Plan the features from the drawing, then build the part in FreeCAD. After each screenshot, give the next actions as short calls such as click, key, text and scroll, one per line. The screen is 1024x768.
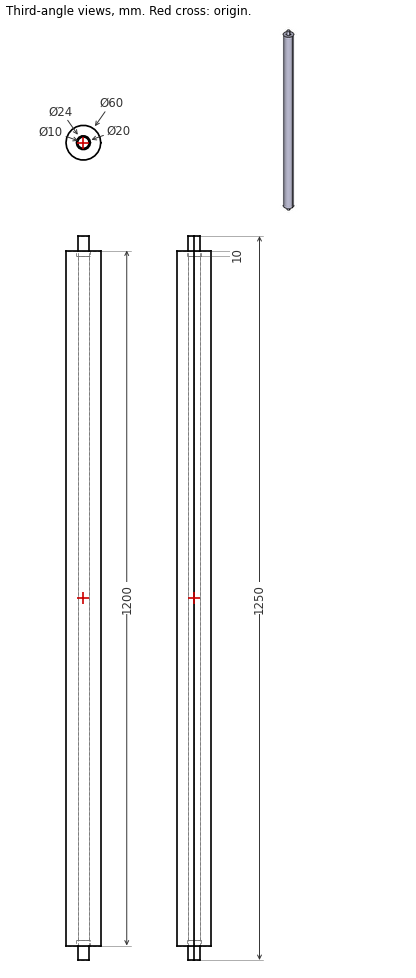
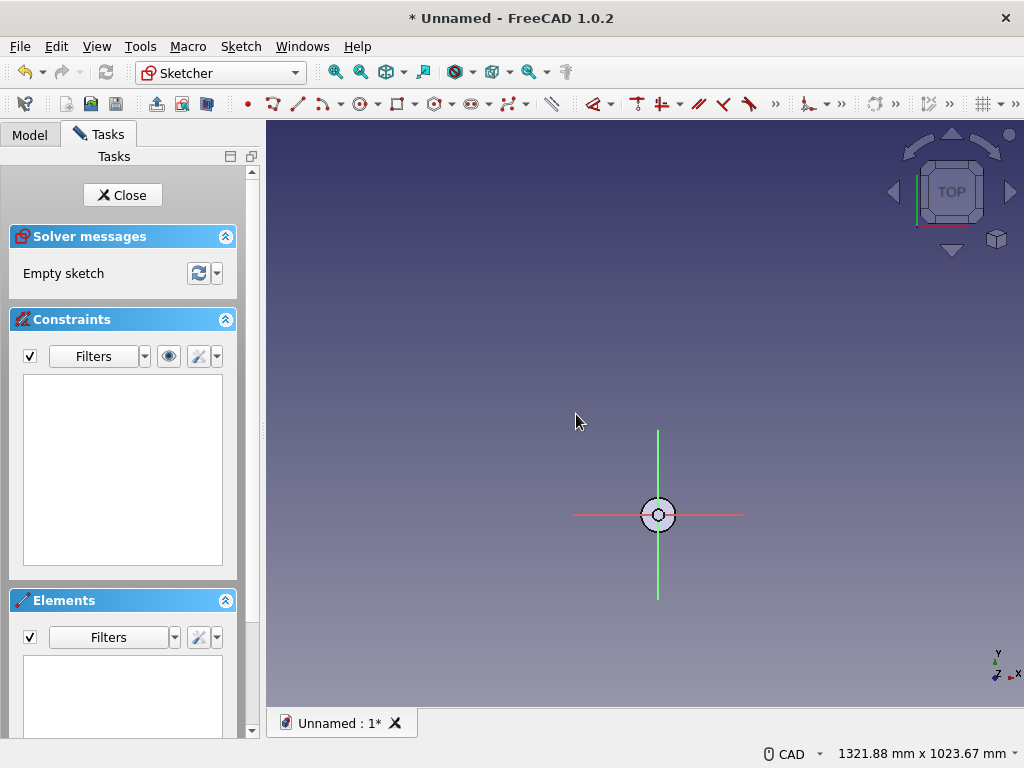
scroll(663, 520, up, 15)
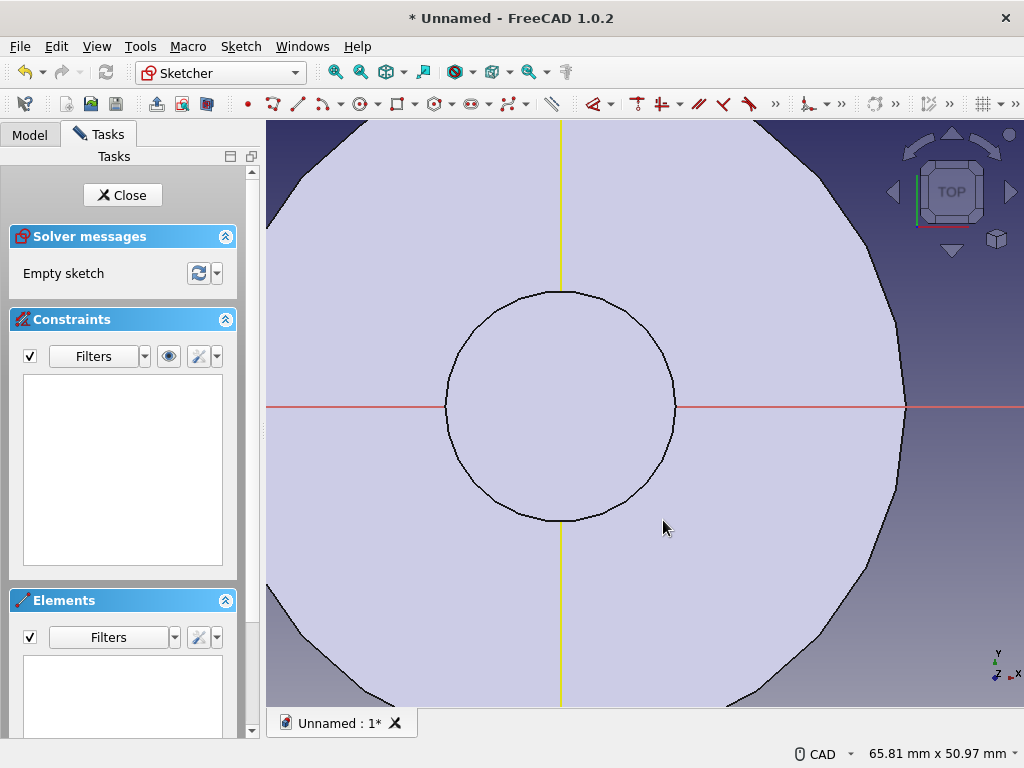
scroll(528, 392, up, 2)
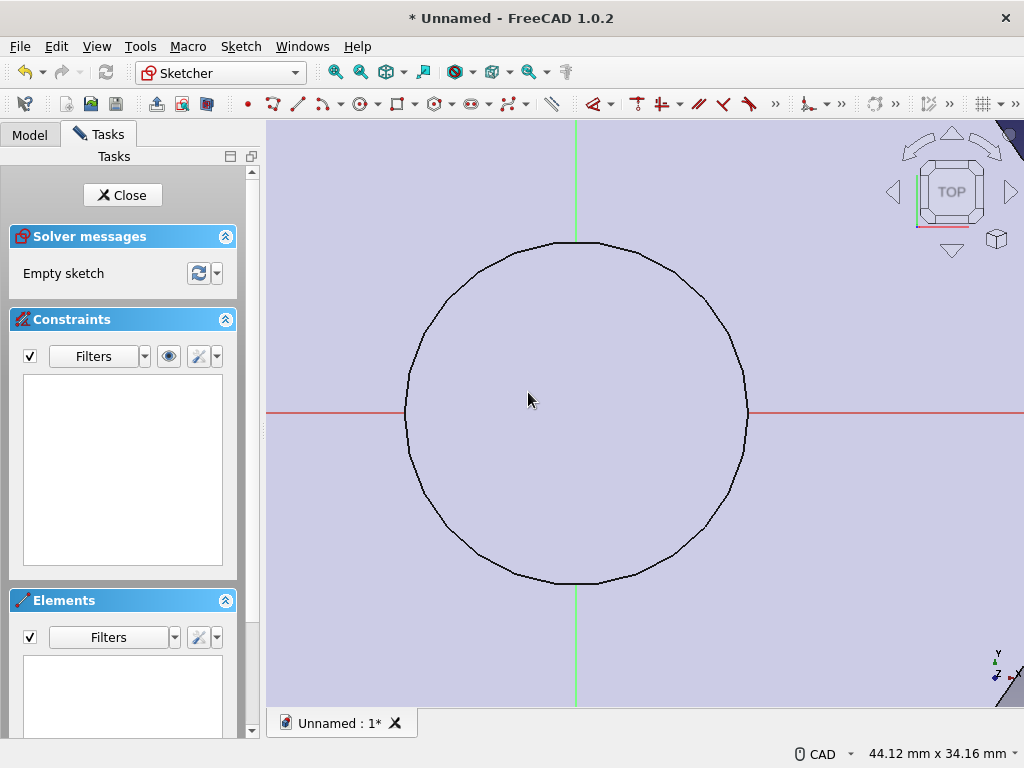
click(360, 104)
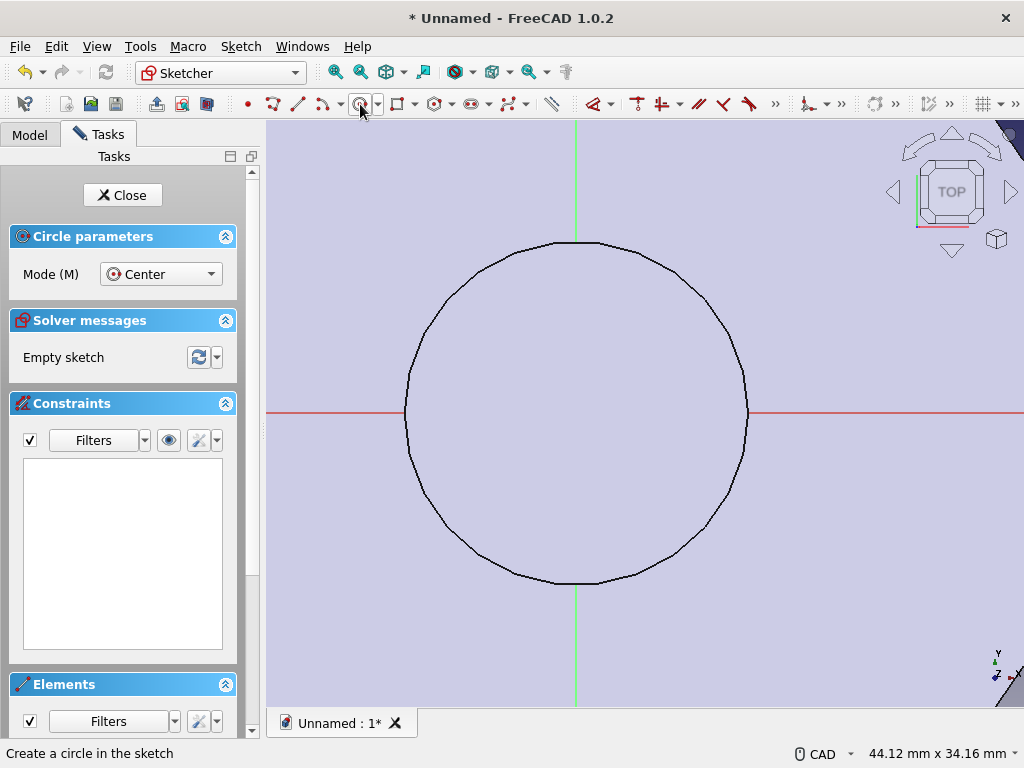
click(576, 413)
click(722, 268)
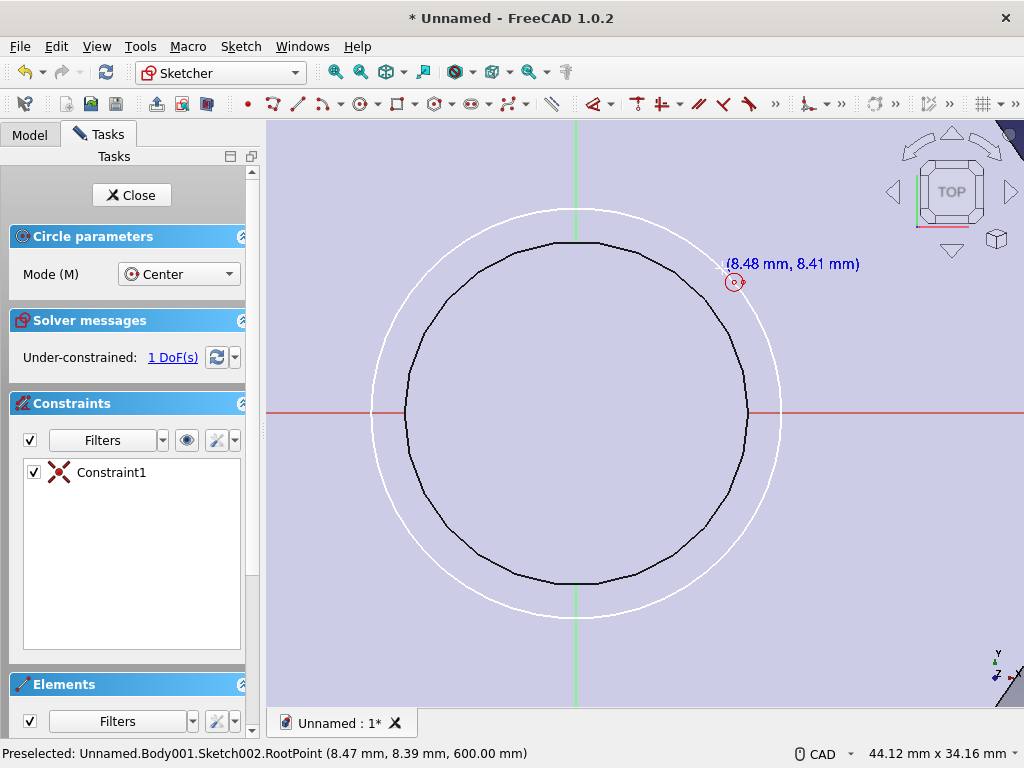
click(576, 413)
click(637, 353)
key(Escape)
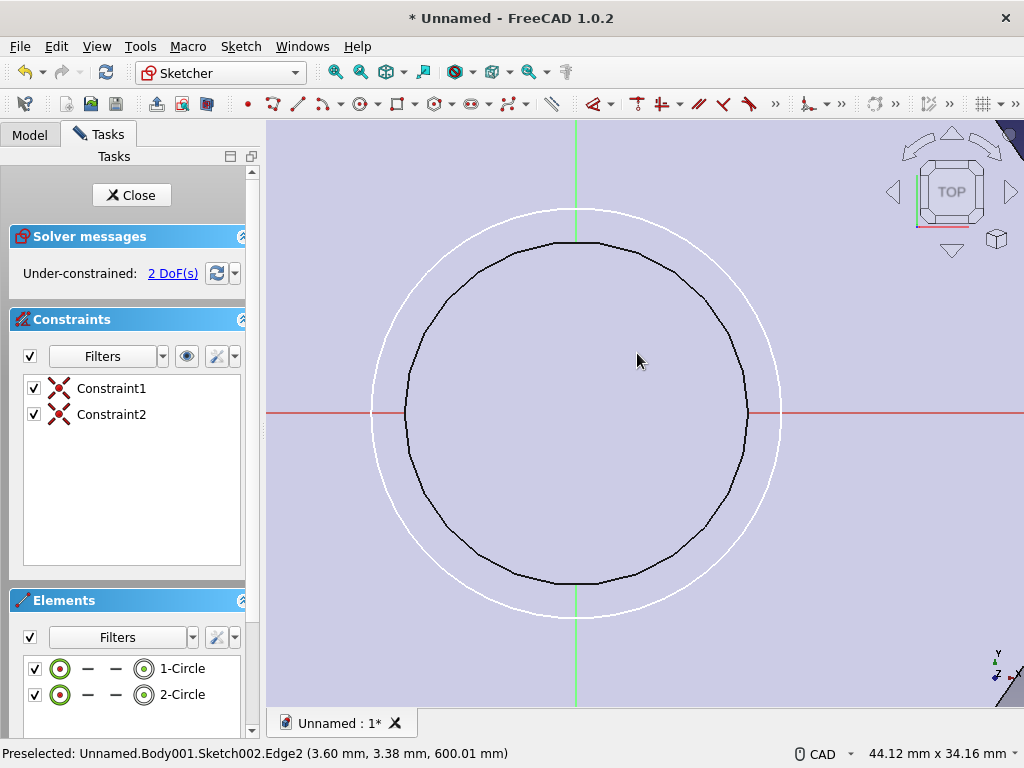
key(d)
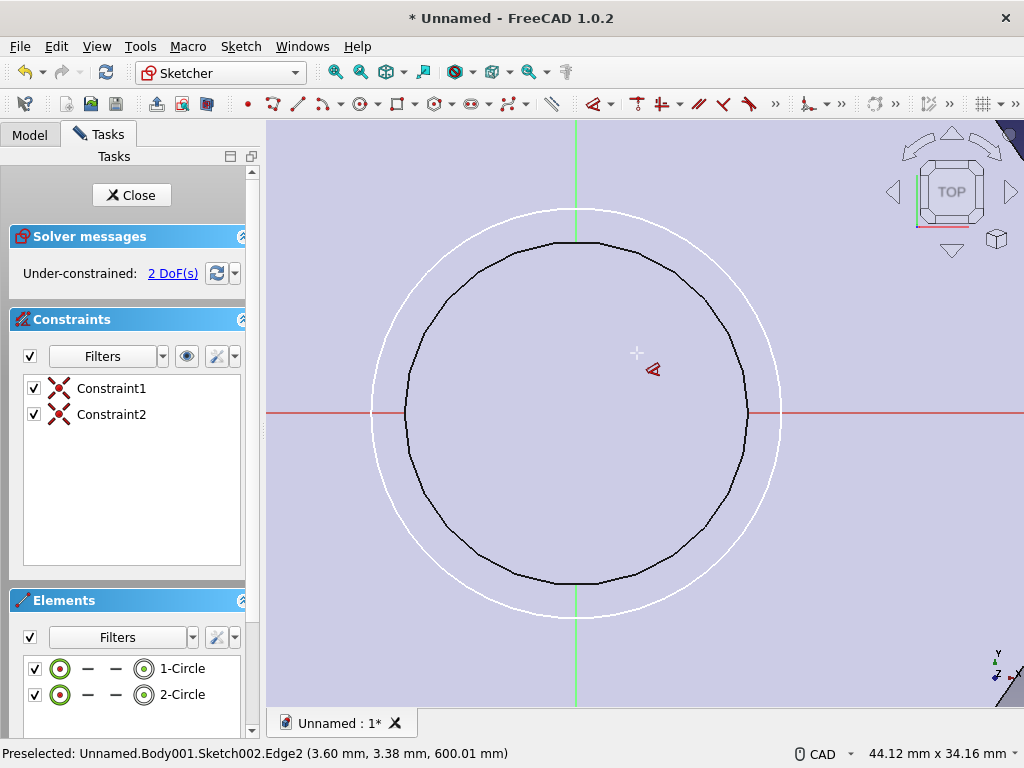
click(721, 268)
click(744, 245)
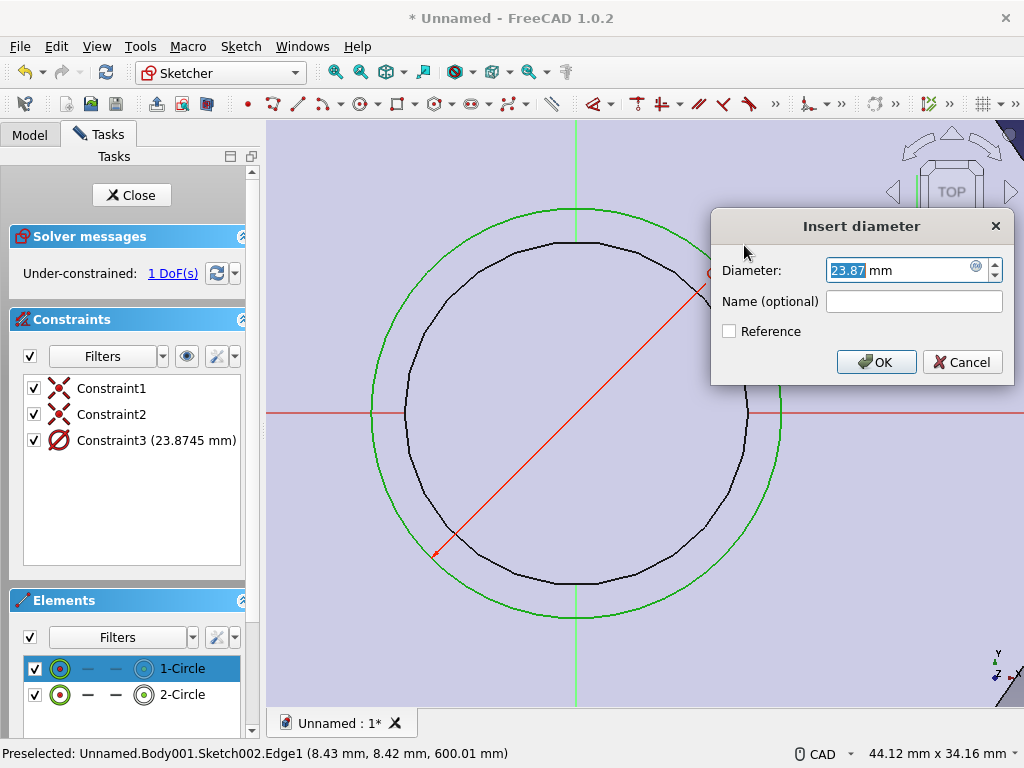
text(24)
key(Return)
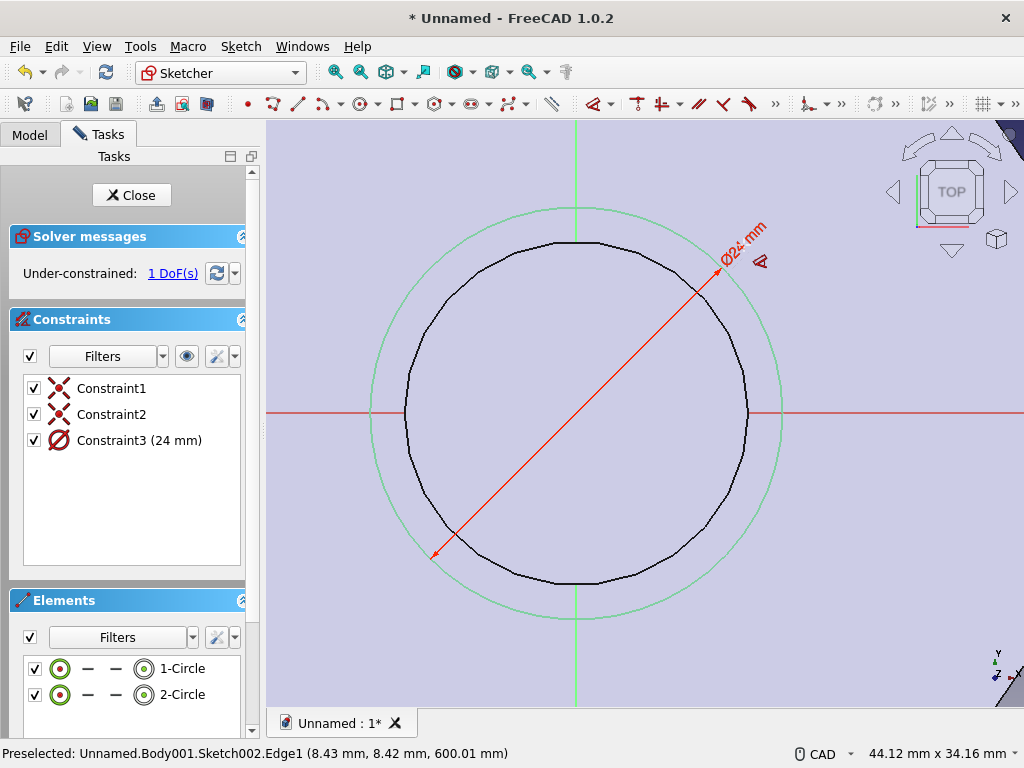
click(636, 353)
click(658, 330)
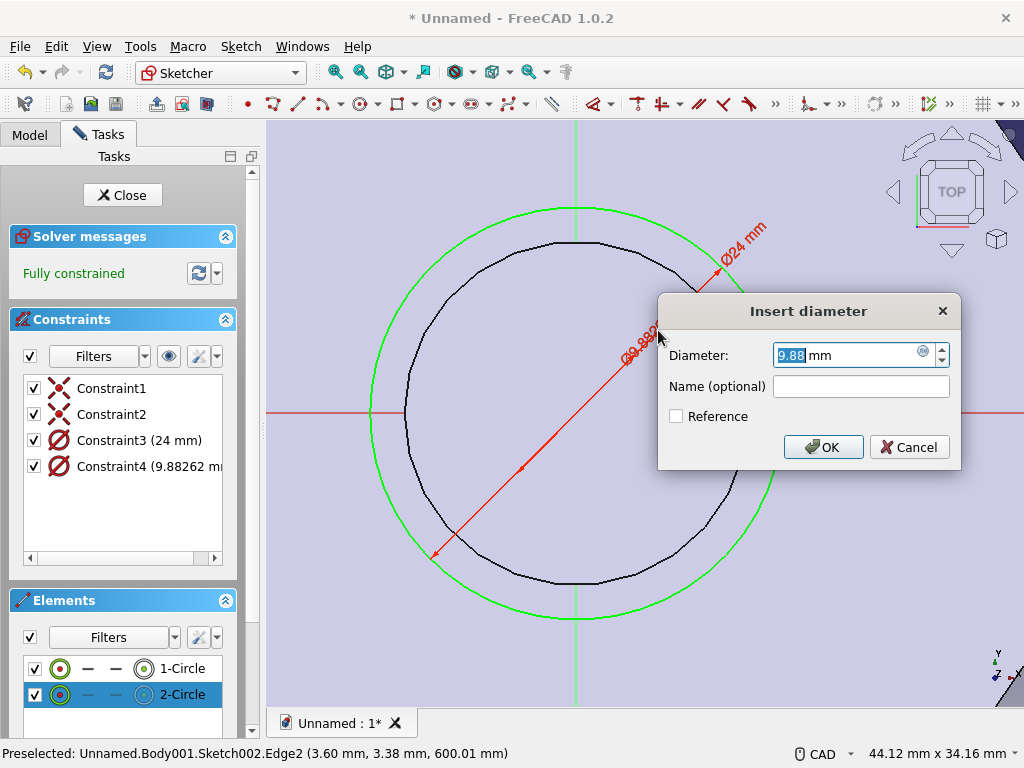
text(10)
key(Return)
key(Escape)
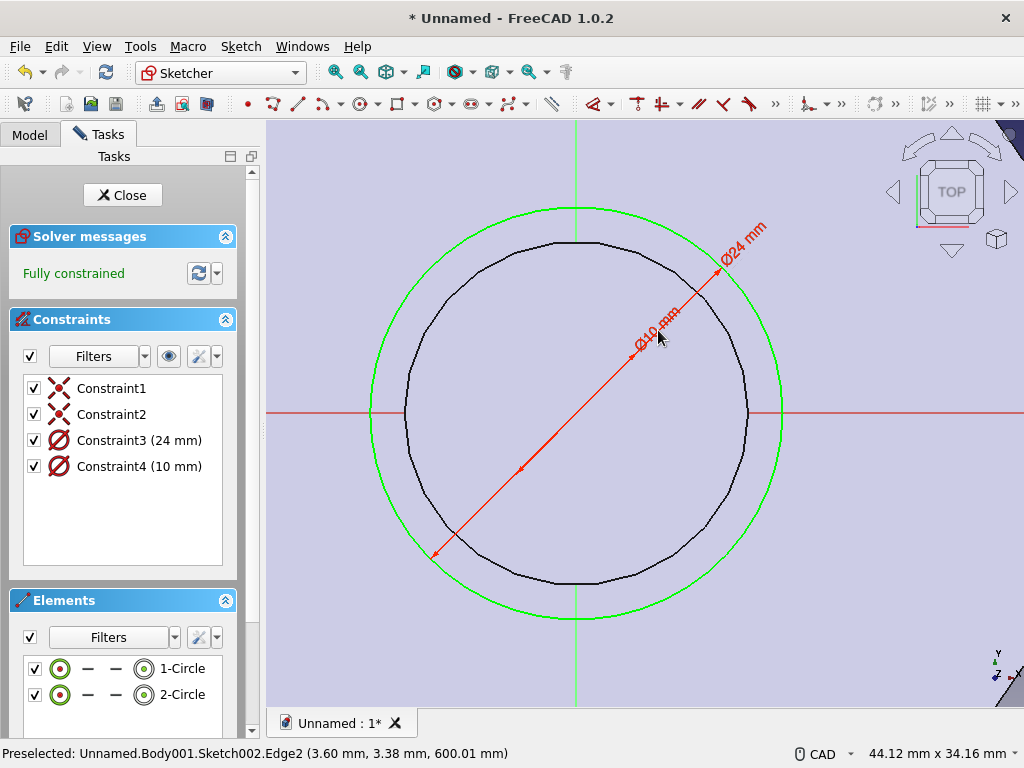
click(123, 195)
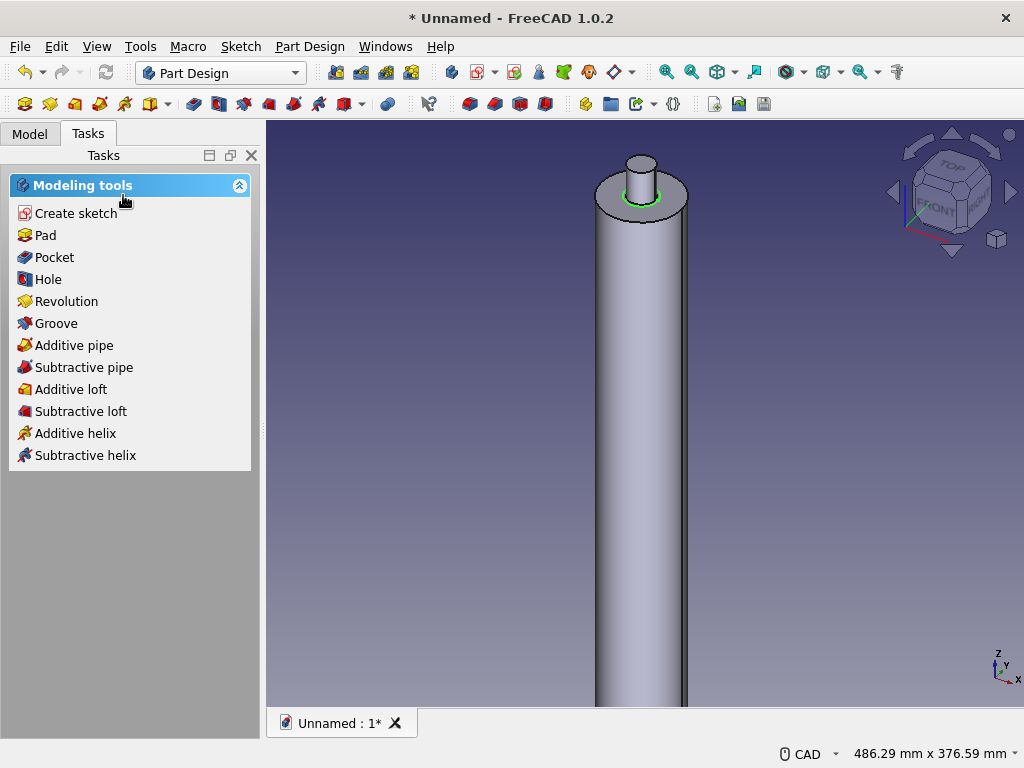
click(194, 104)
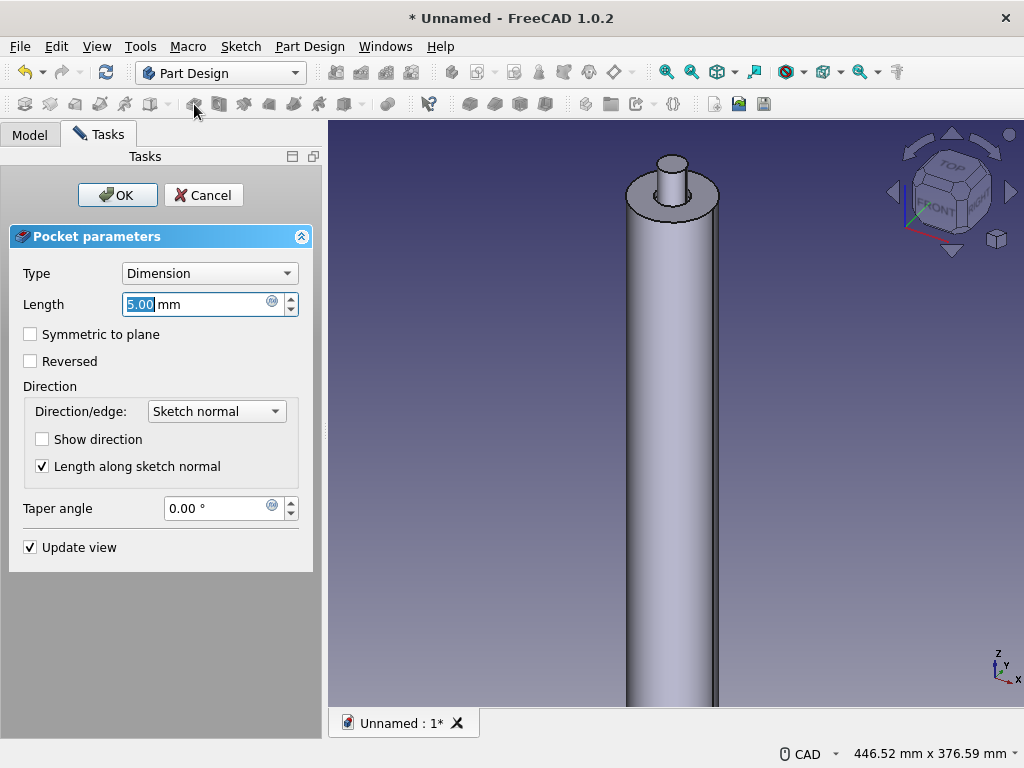
text(10)
key(Tab)